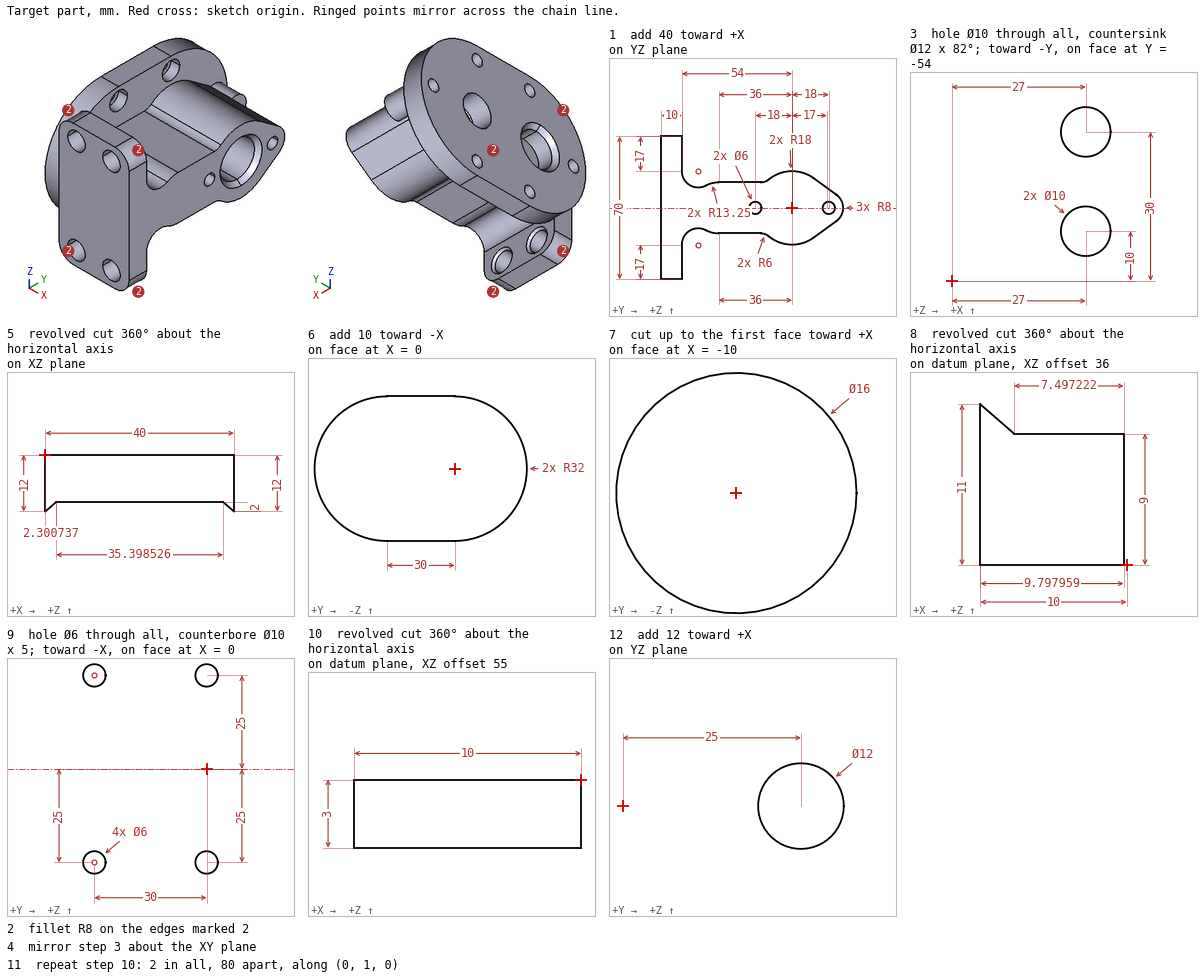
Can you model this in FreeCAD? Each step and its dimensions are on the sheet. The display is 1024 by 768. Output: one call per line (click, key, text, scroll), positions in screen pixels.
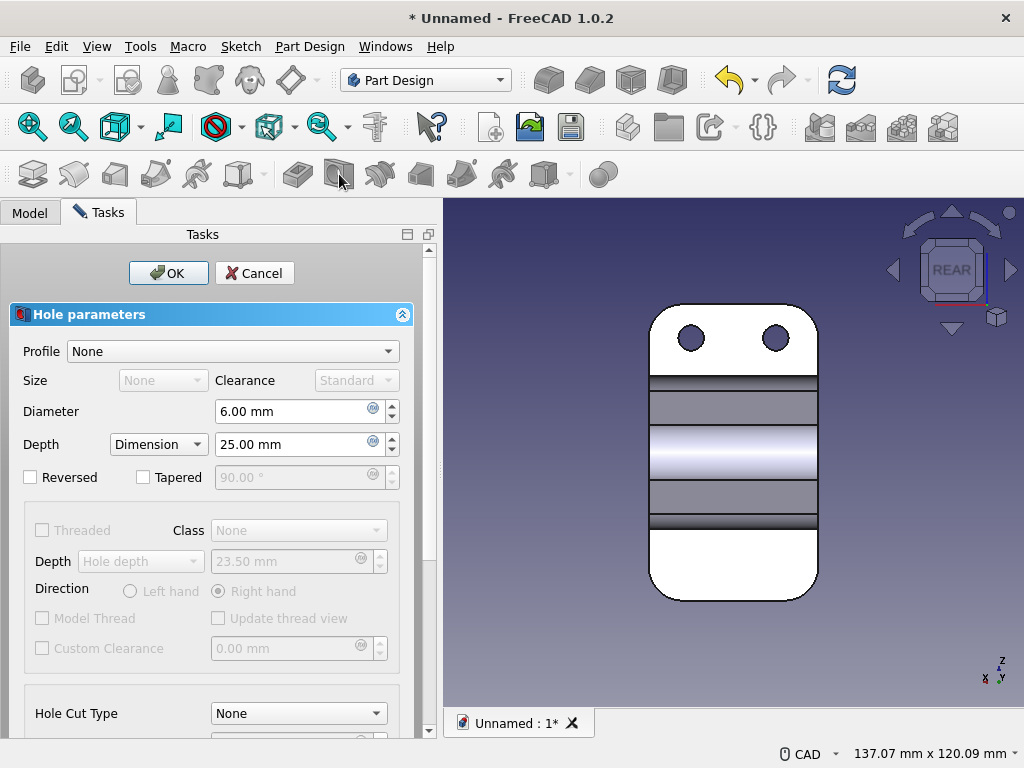
triple_click(300, 412)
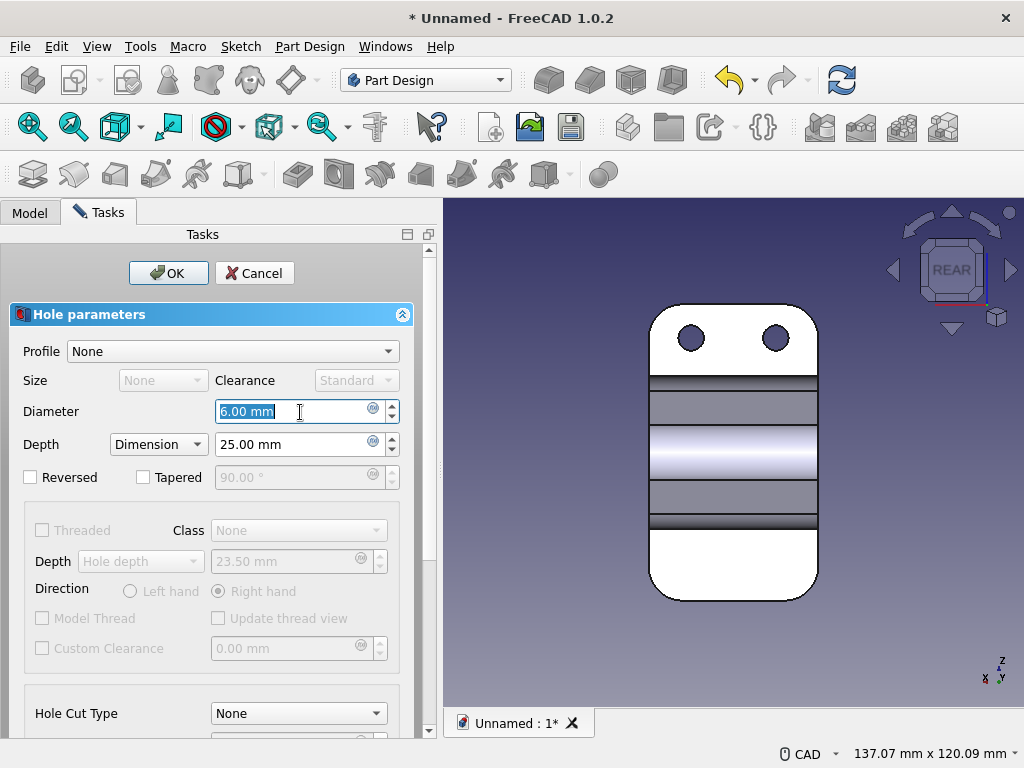
text(10)
key(Tab)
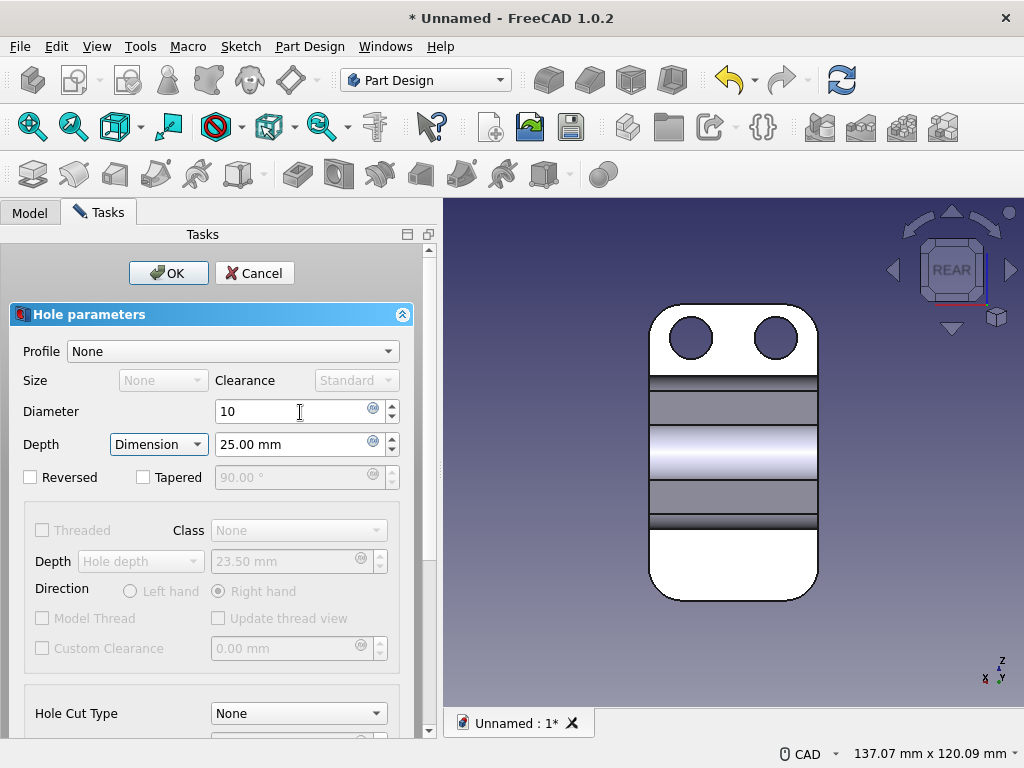
click(160, 444)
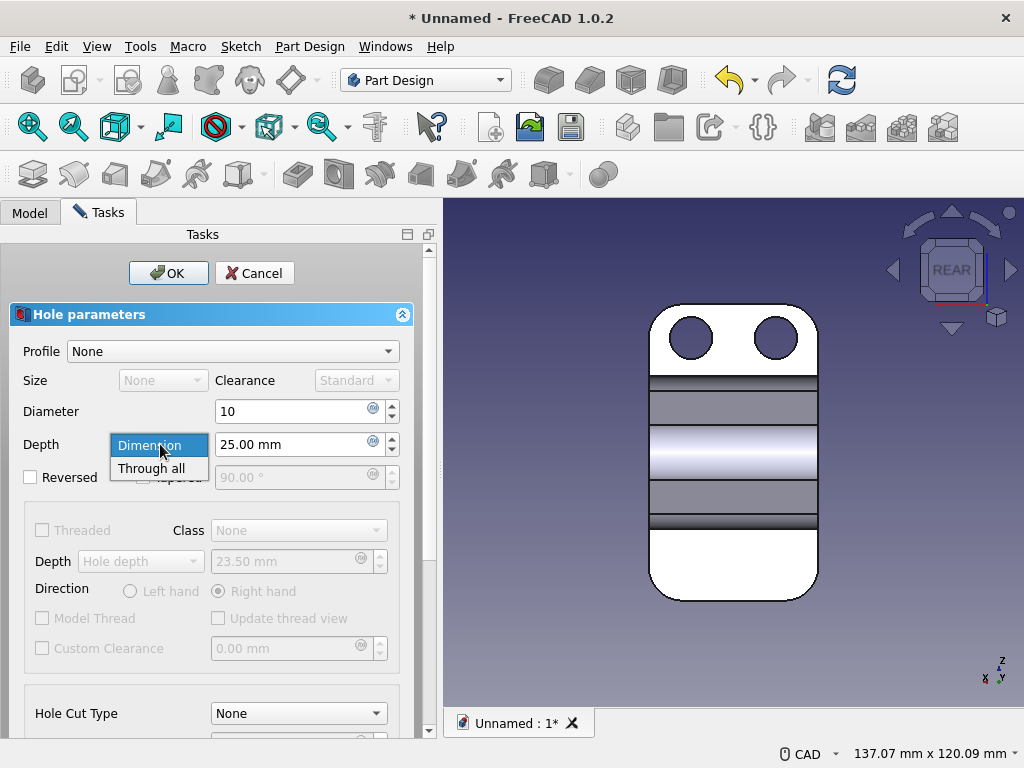
click(158, 468)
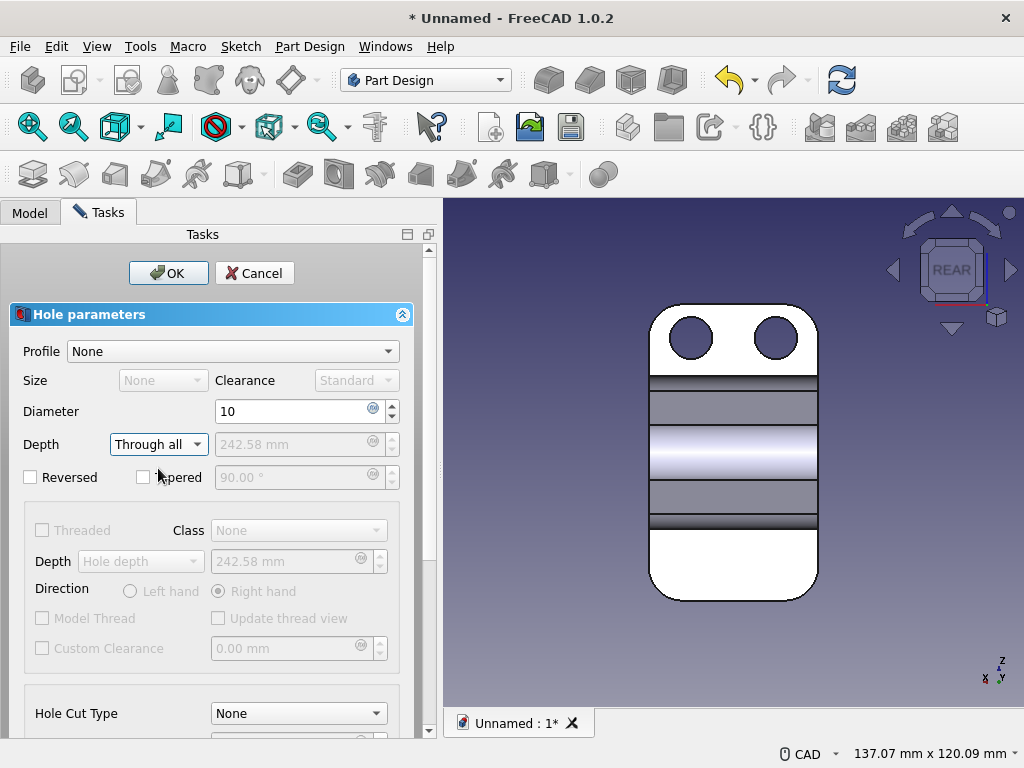
click(300, 714)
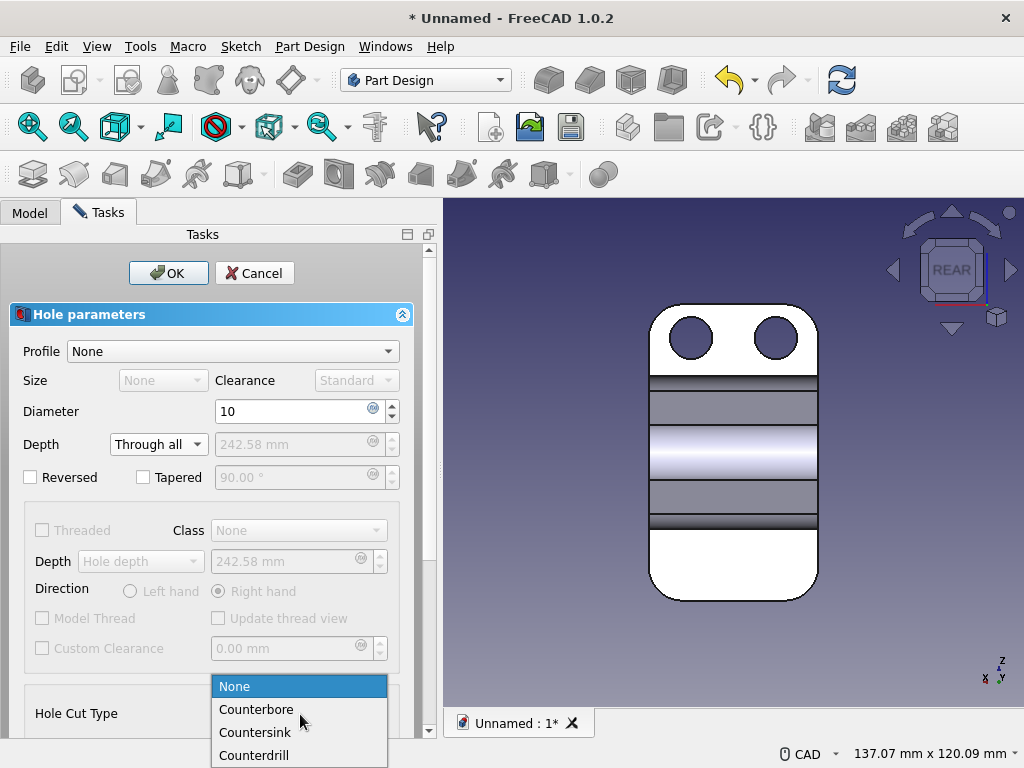
click(298, 732)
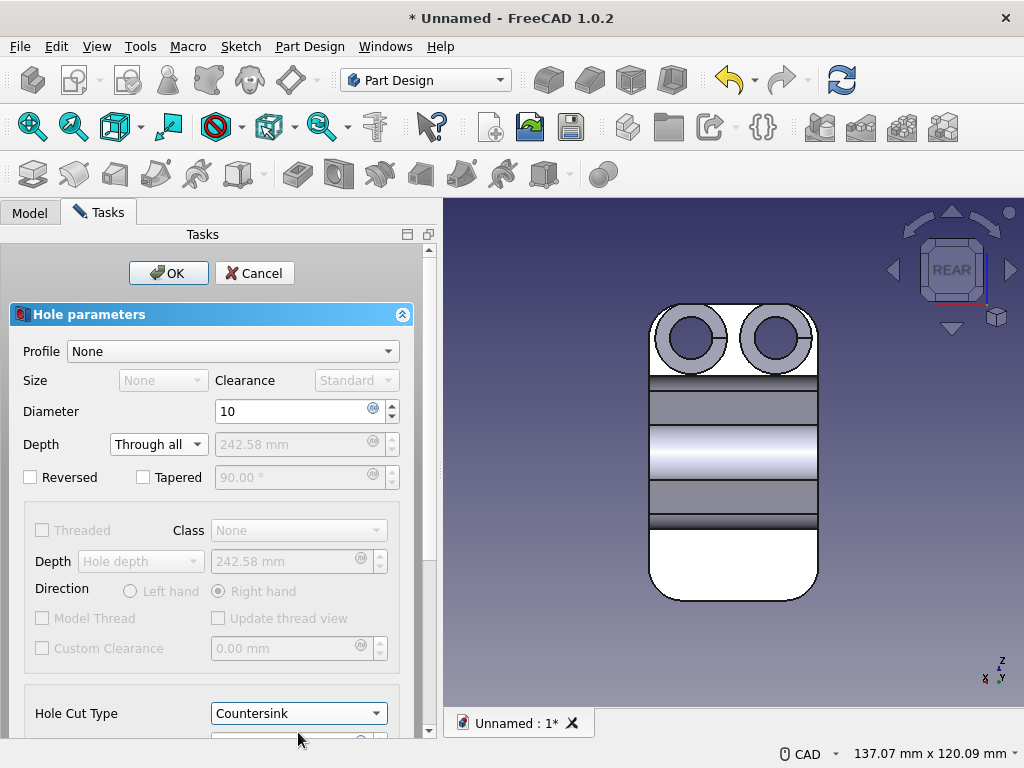
scroll(429, 491, down, 3)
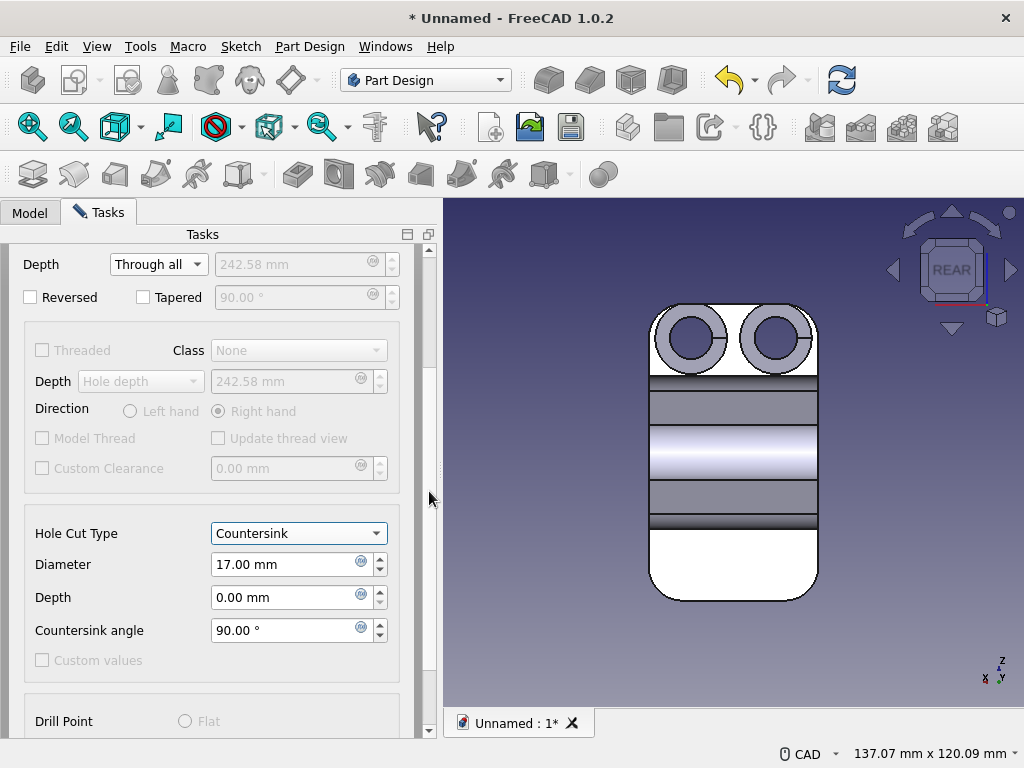
triple_click(292, 630)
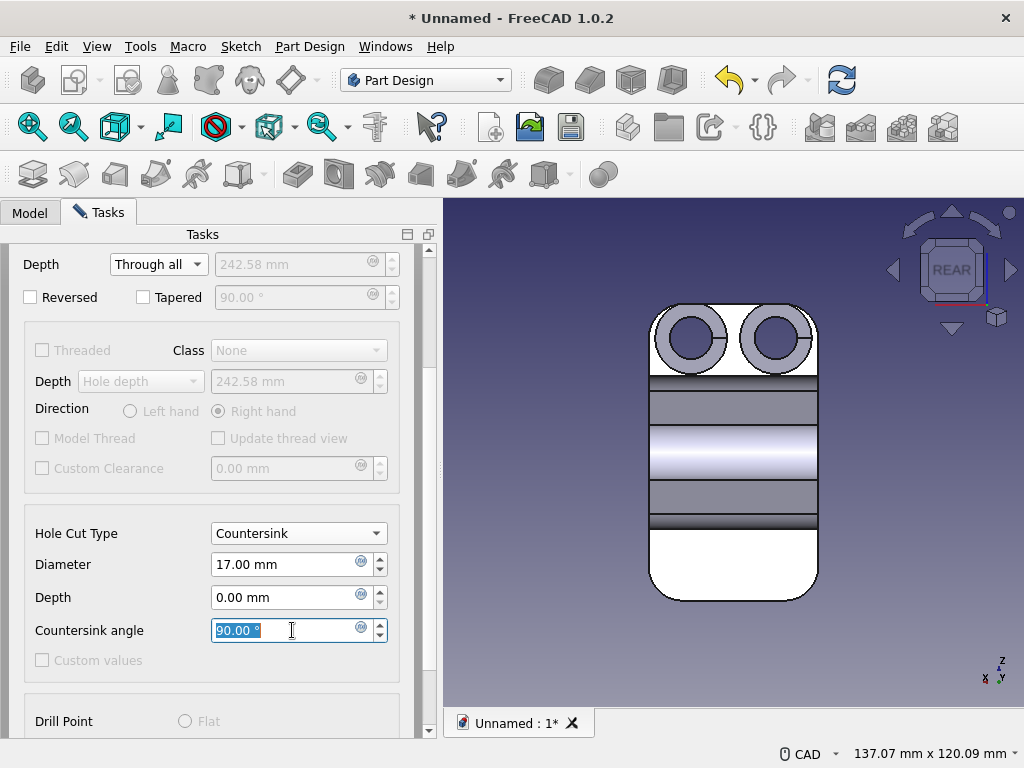
text(82)
key(Tab)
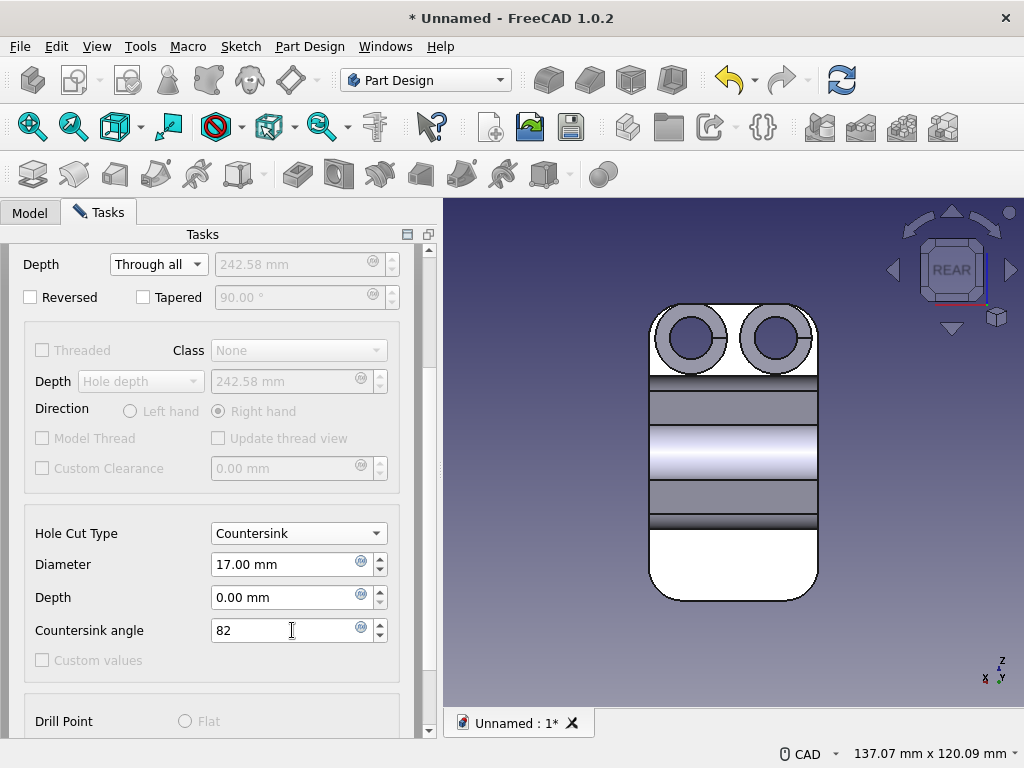
triple_click(292, 564)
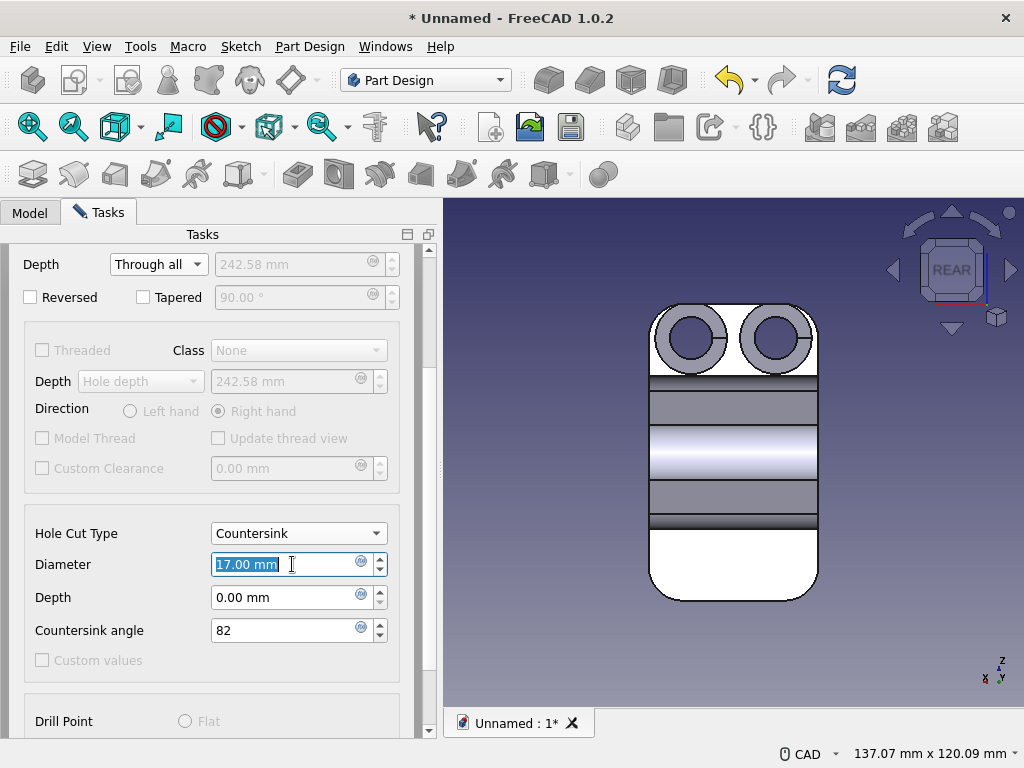
text(12)
key(Tab)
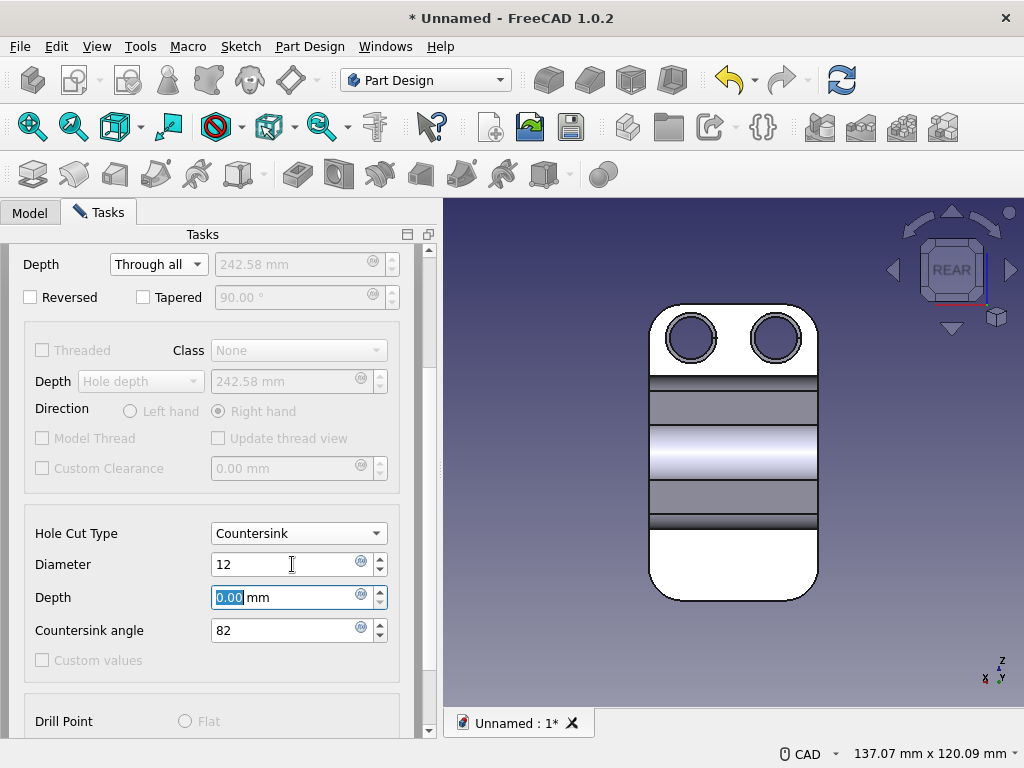
scroll(429, 491, up, 4)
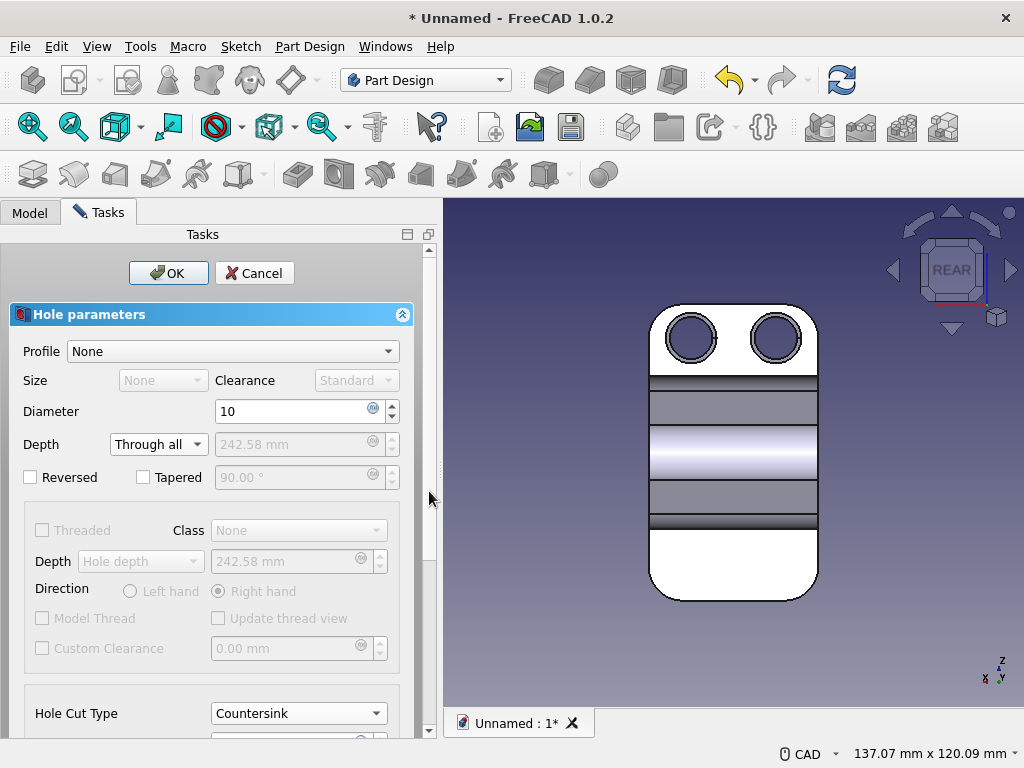
click(169, 273)